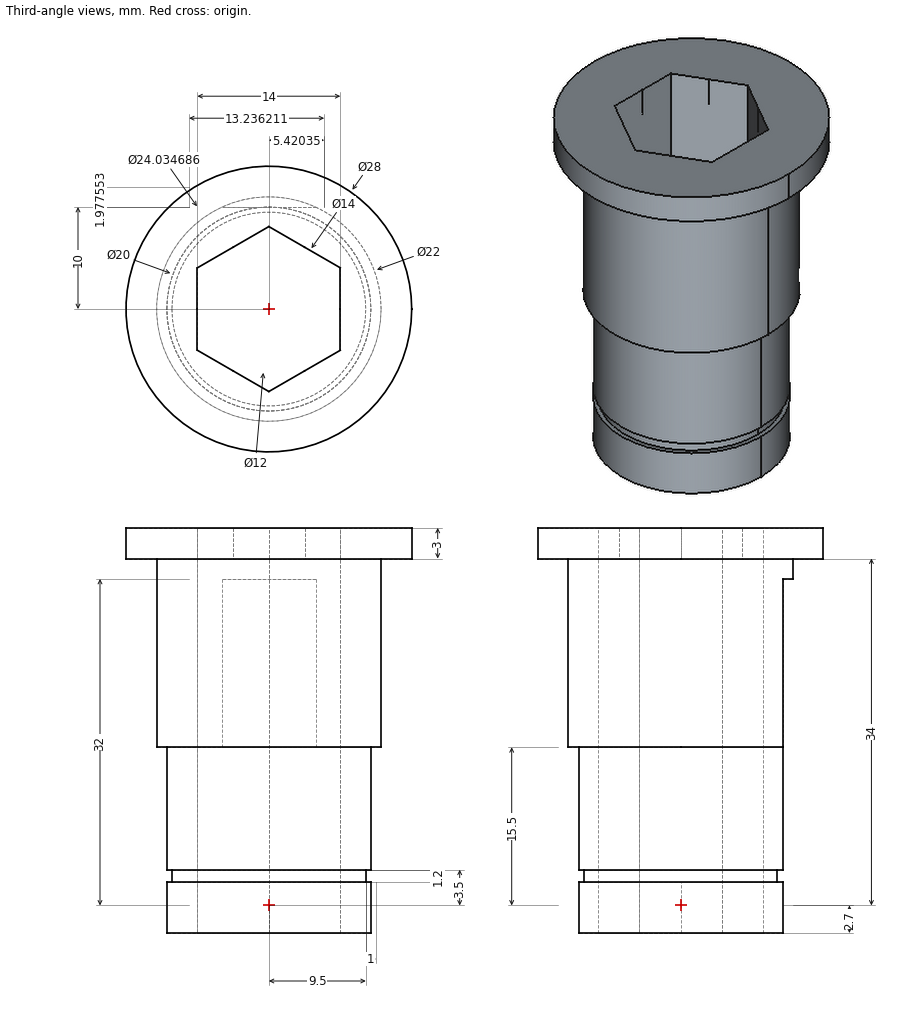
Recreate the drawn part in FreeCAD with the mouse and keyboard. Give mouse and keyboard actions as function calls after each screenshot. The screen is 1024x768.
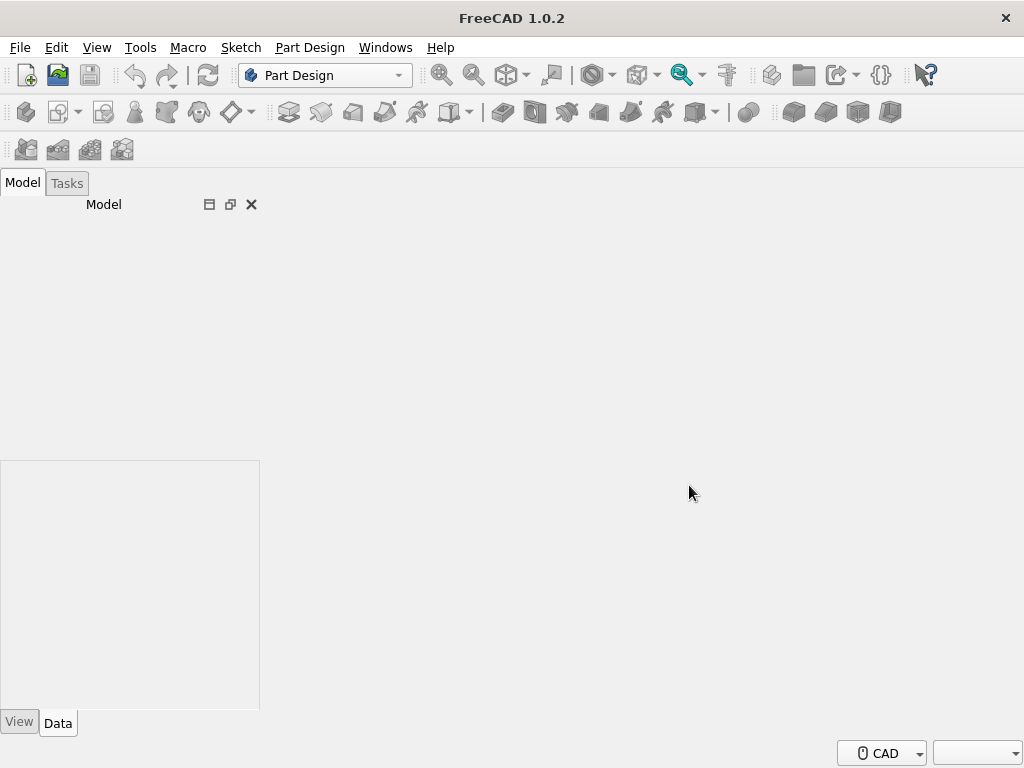
click(26, 76)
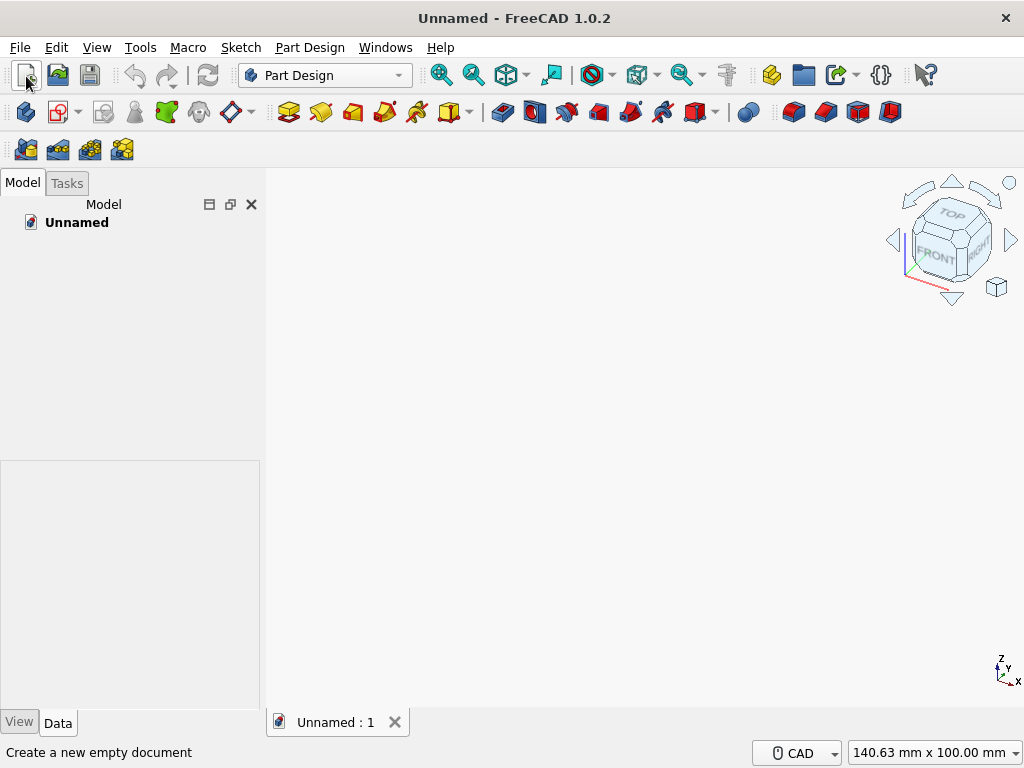
click(58, 112)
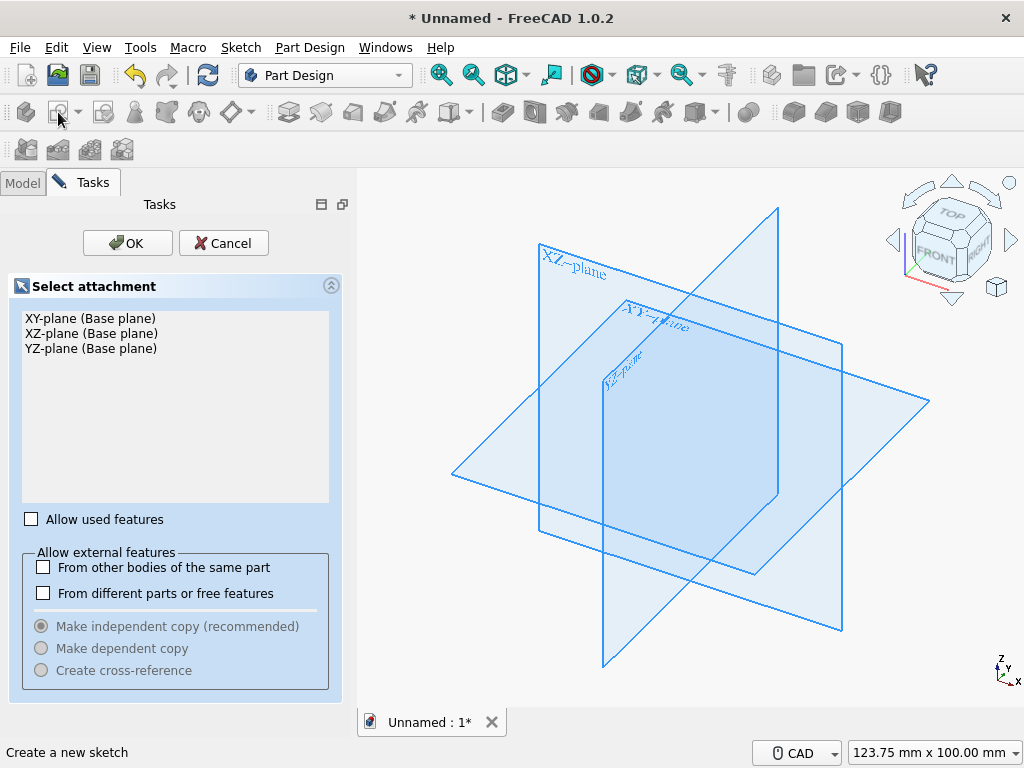
click(82, 318)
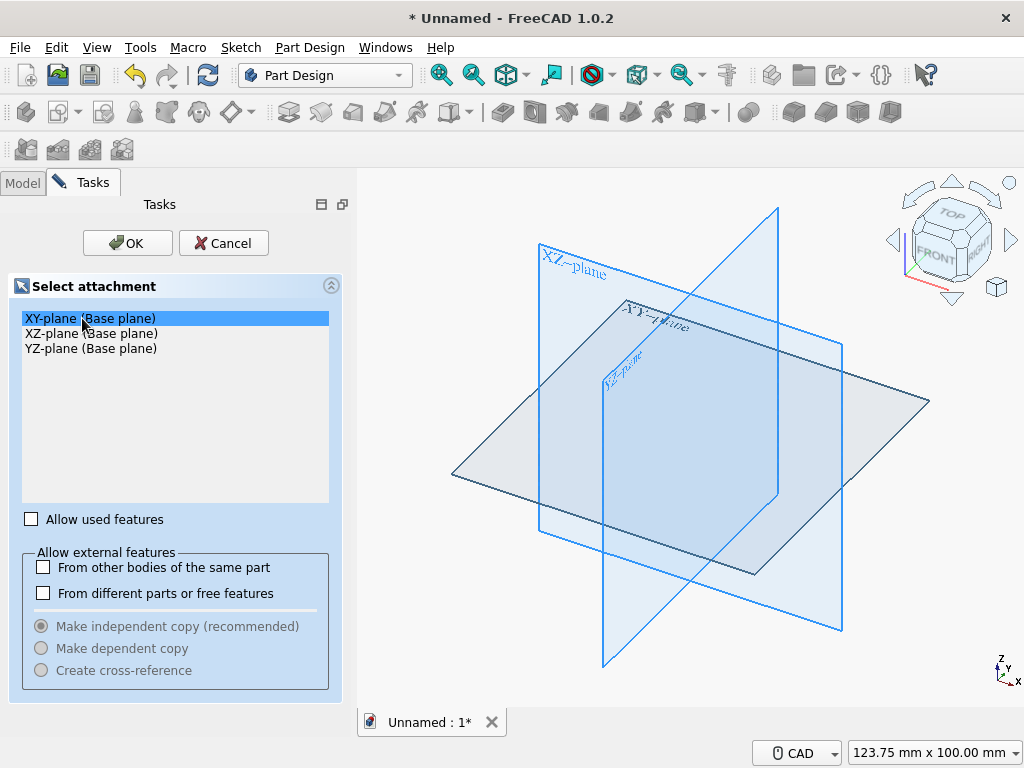
click(128, 243)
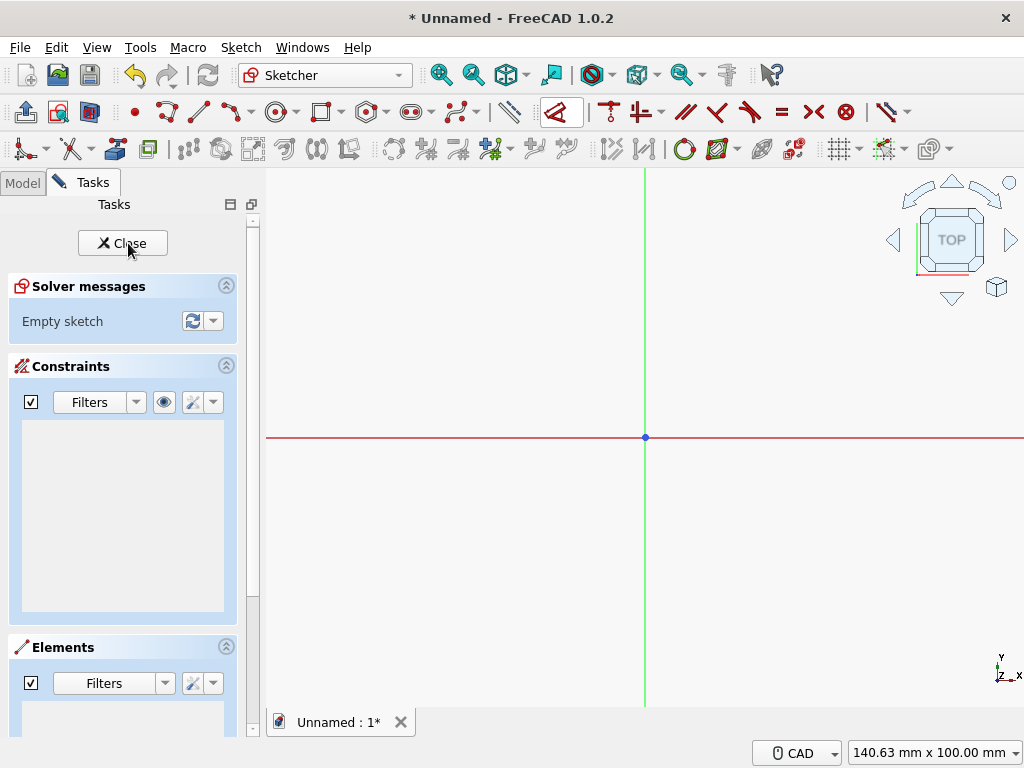
scroll(685, 438, up, 5)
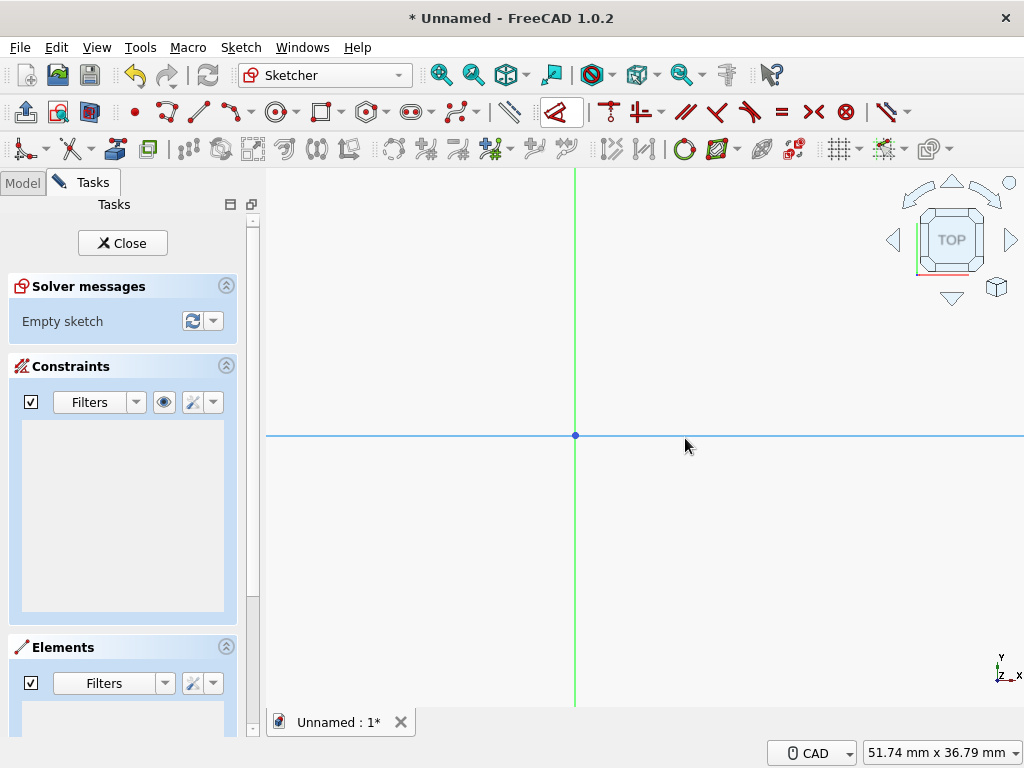
click(276, 112)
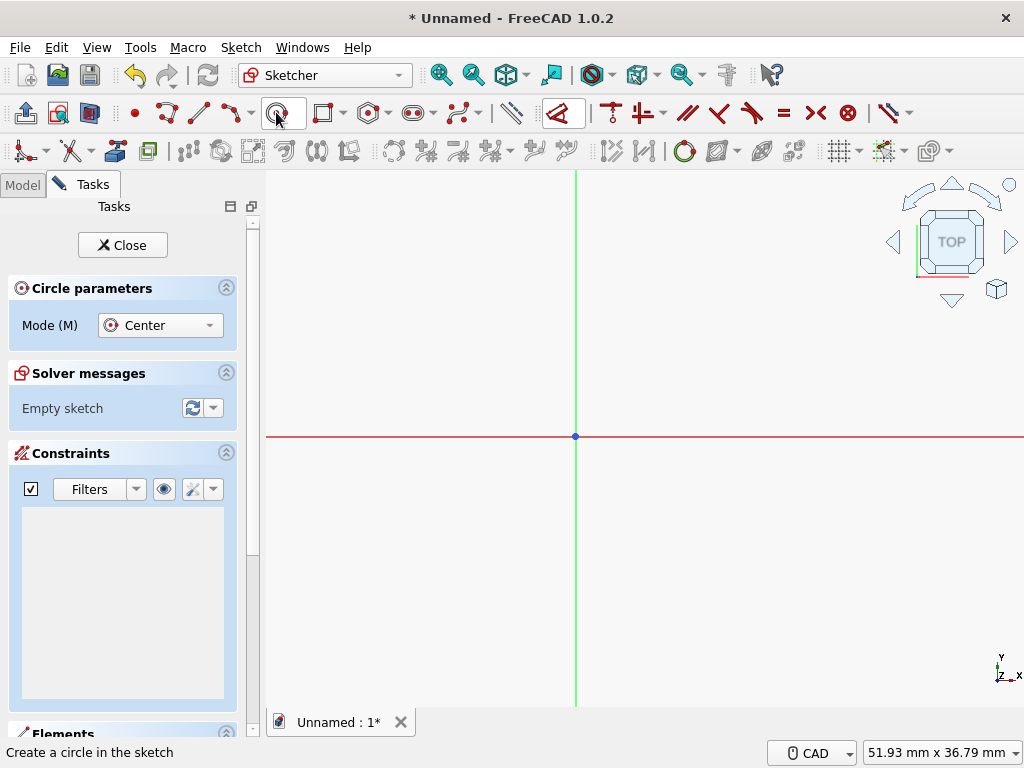
click(576, 437)
click(689, 323)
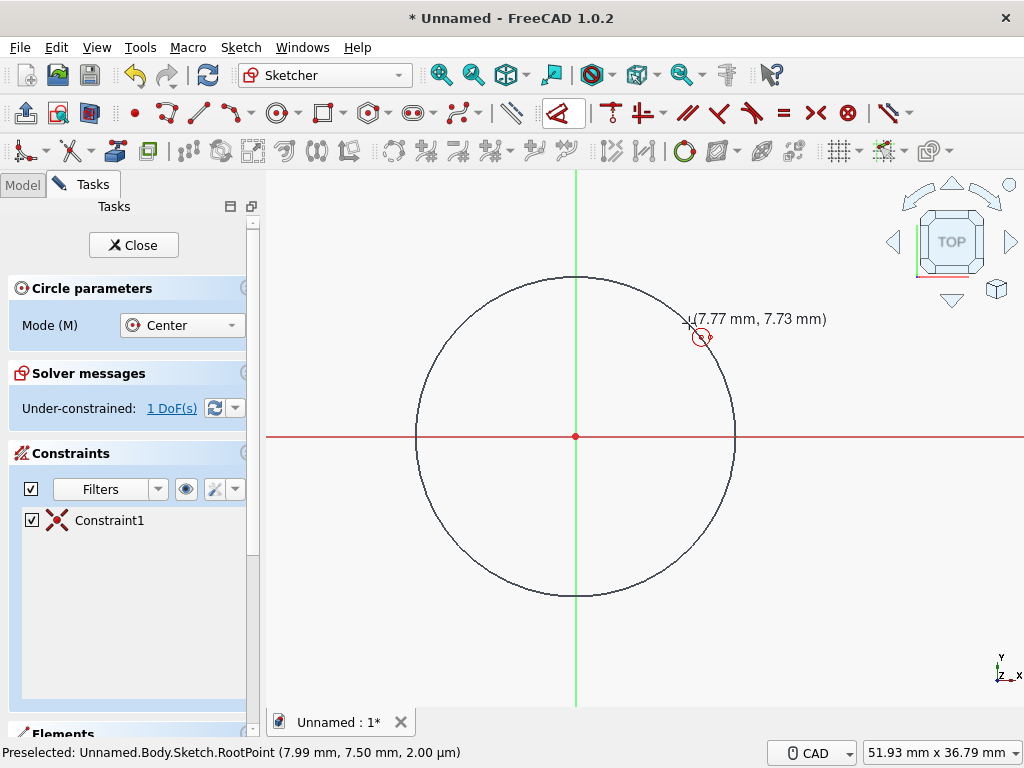
click(576, 437)
click(638, 375)
key(Escape)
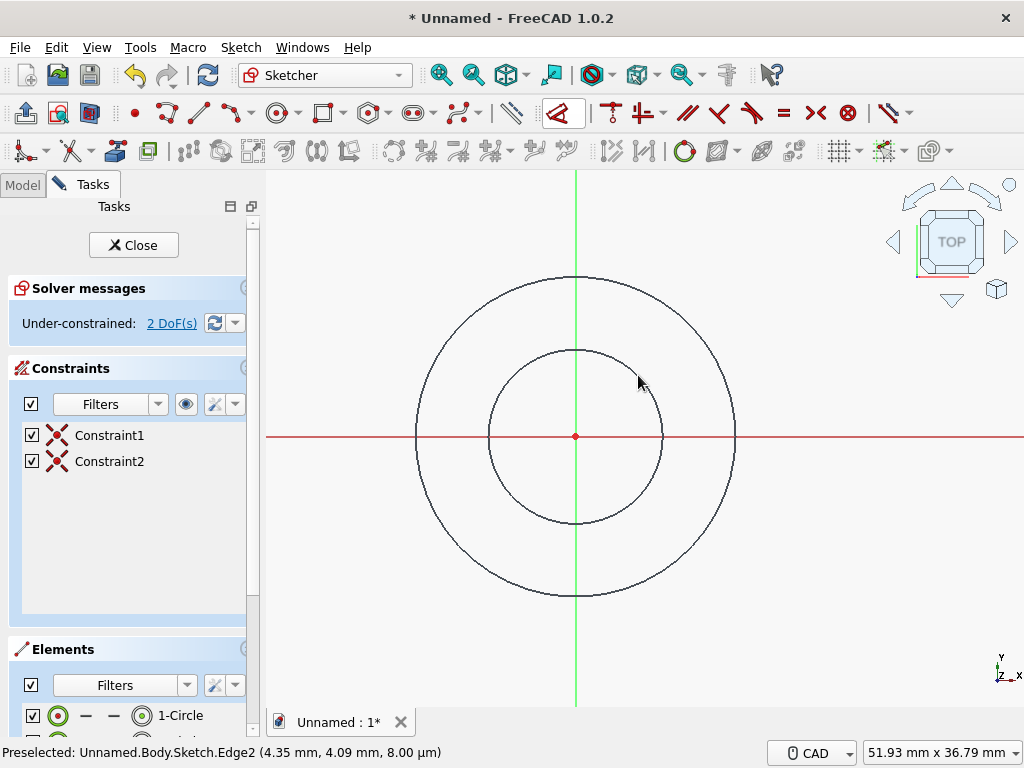
click(558, 114)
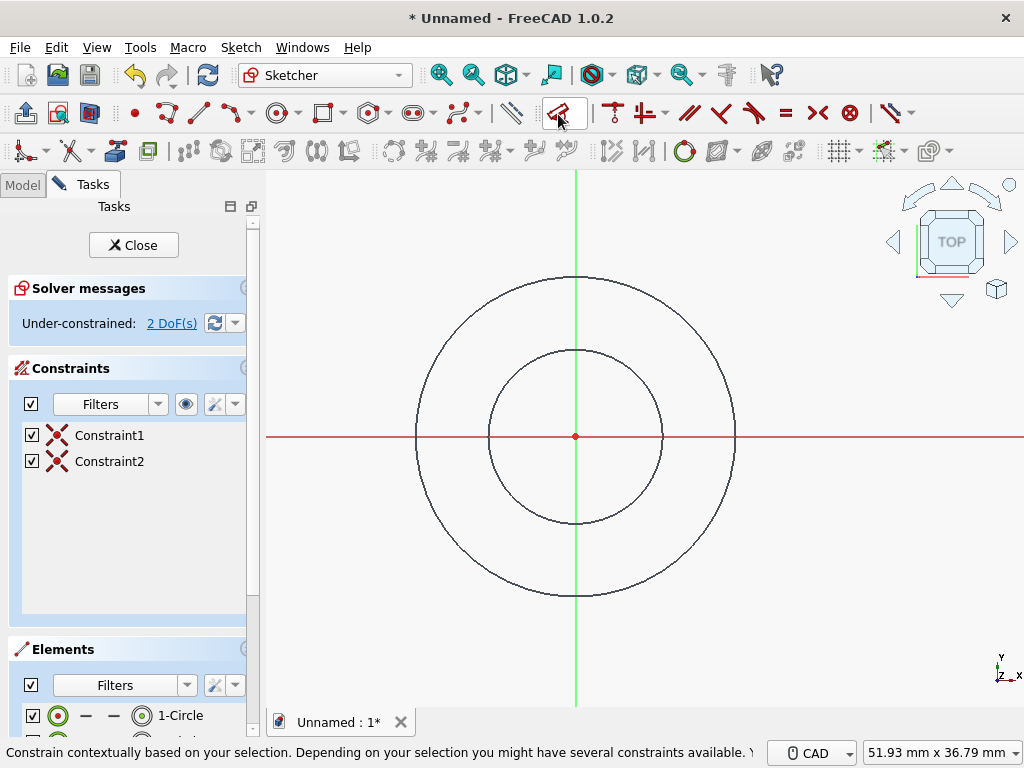
click(688, 323)
click(710, 300)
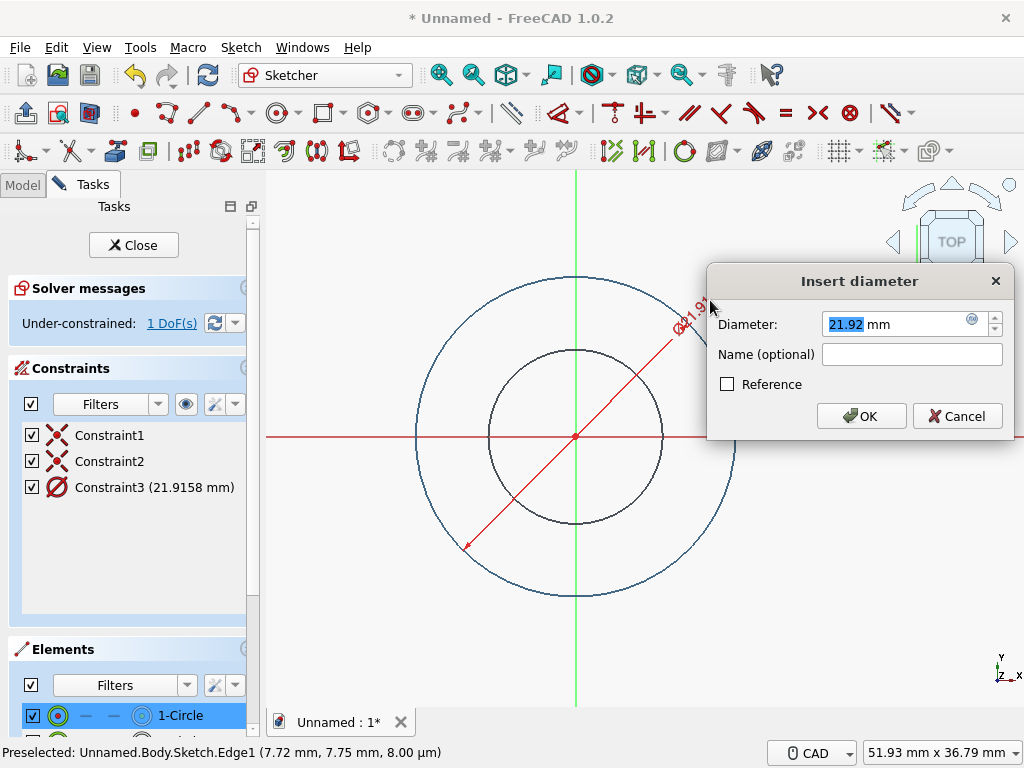
text(22)
key(Return)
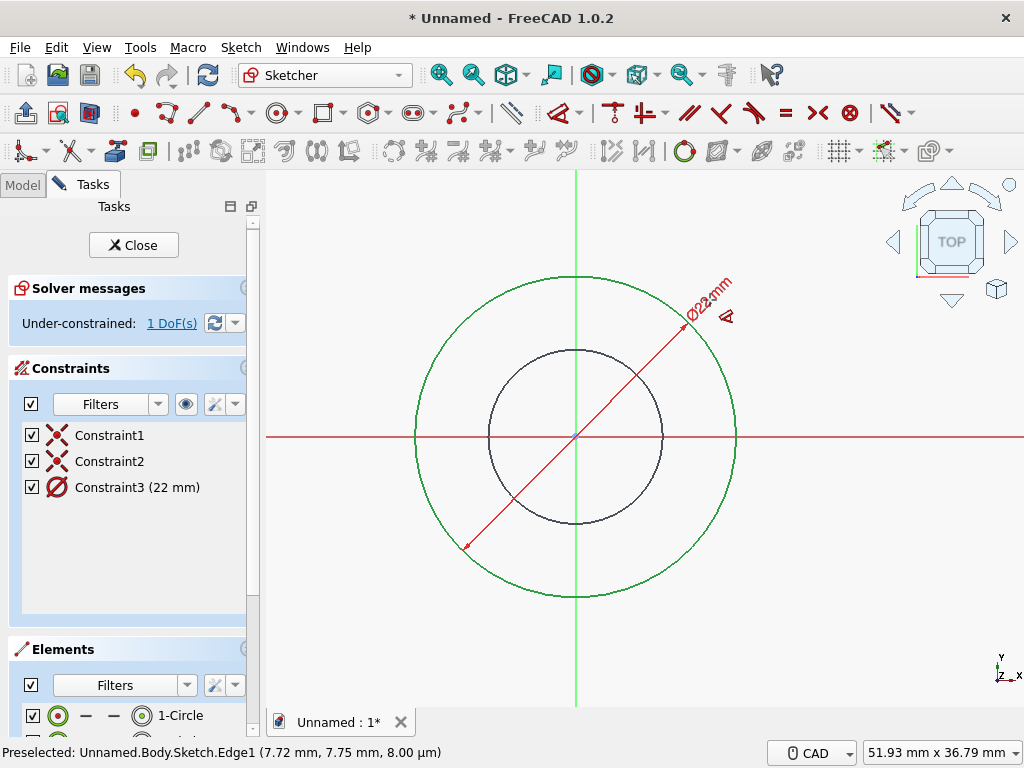
click(637, 375)
click(660, 352)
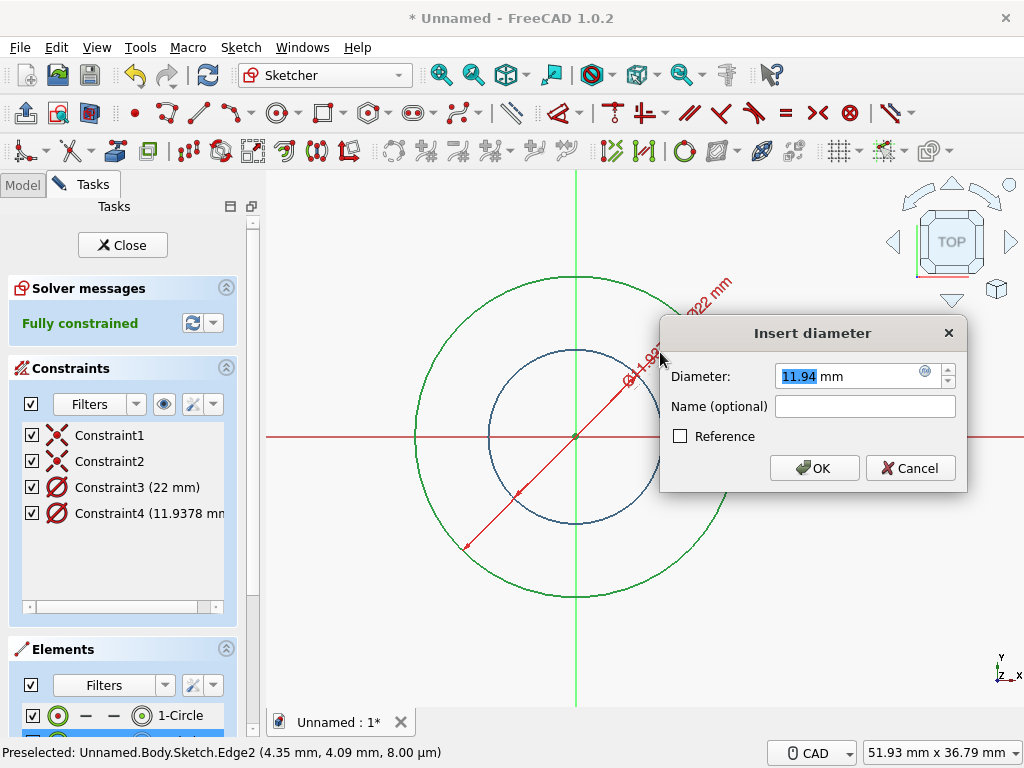
text(12)
key(Return)
key(Escape)